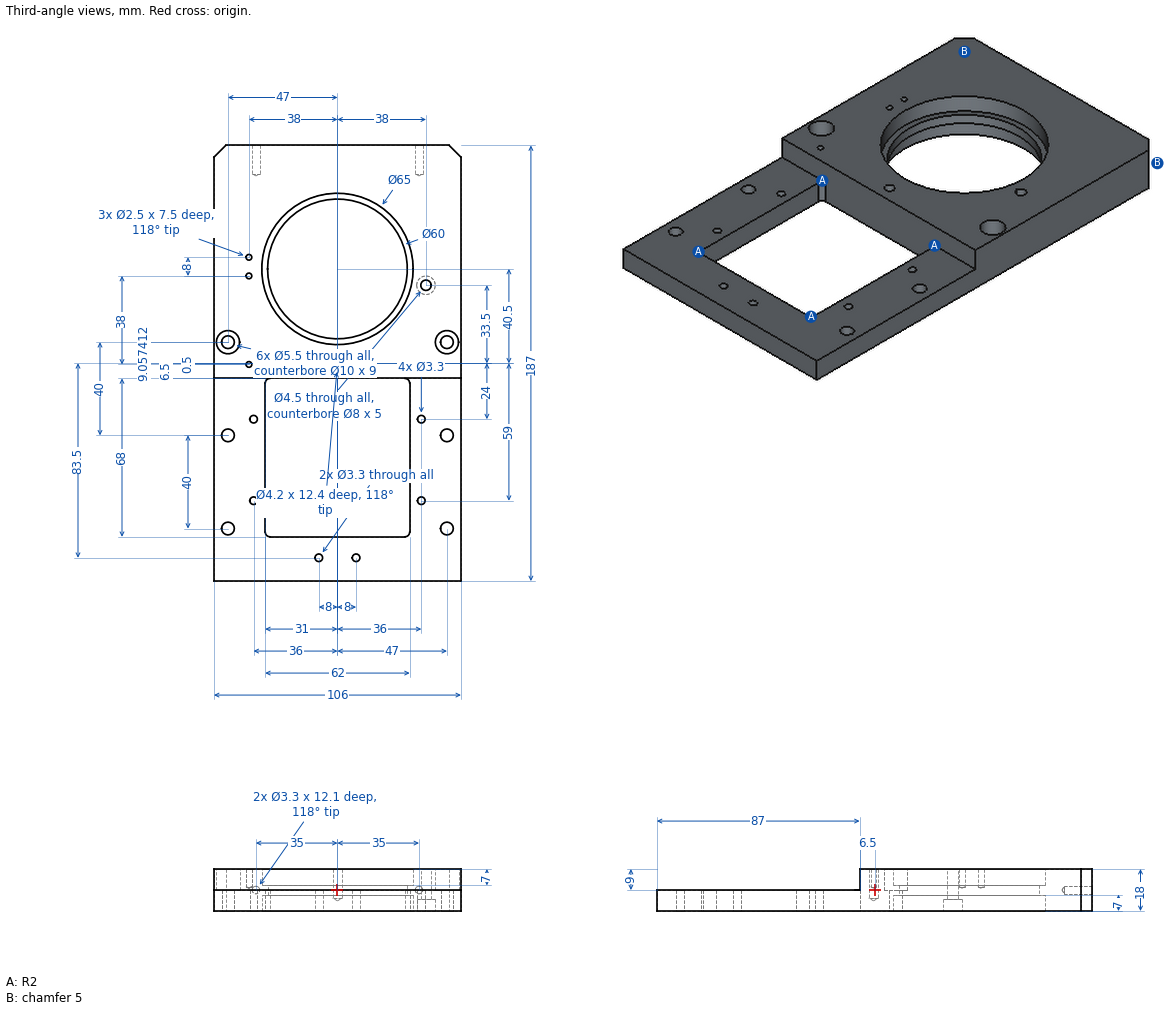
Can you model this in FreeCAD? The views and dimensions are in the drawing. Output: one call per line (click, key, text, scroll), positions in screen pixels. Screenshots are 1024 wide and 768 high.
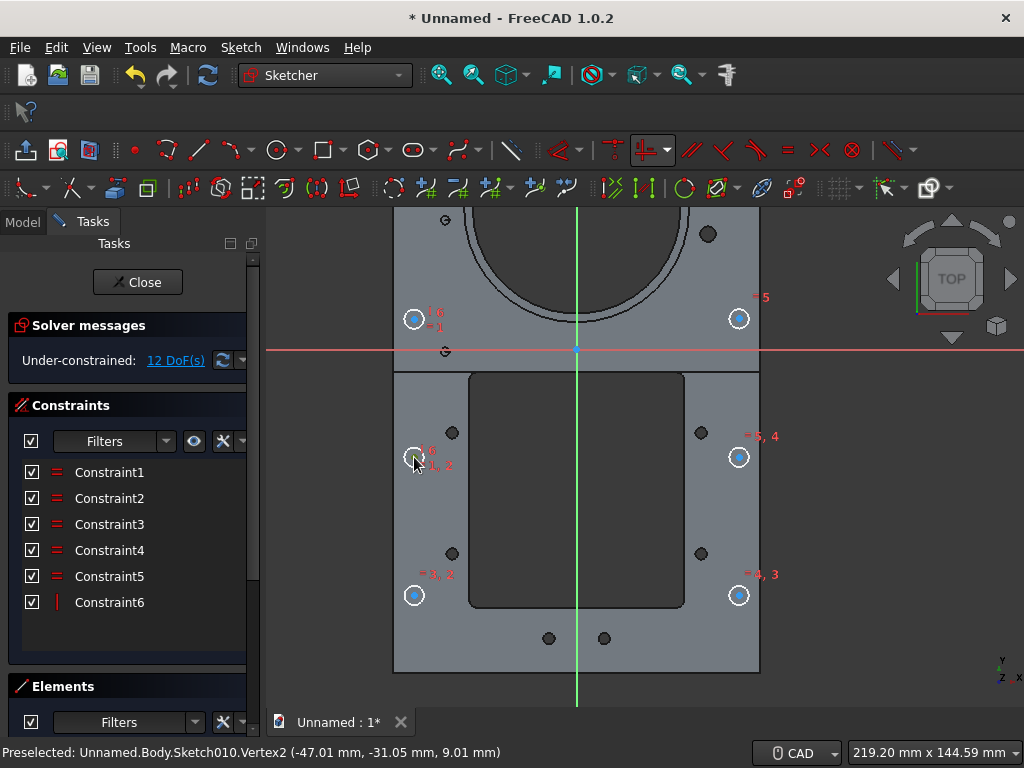
click(414, 595)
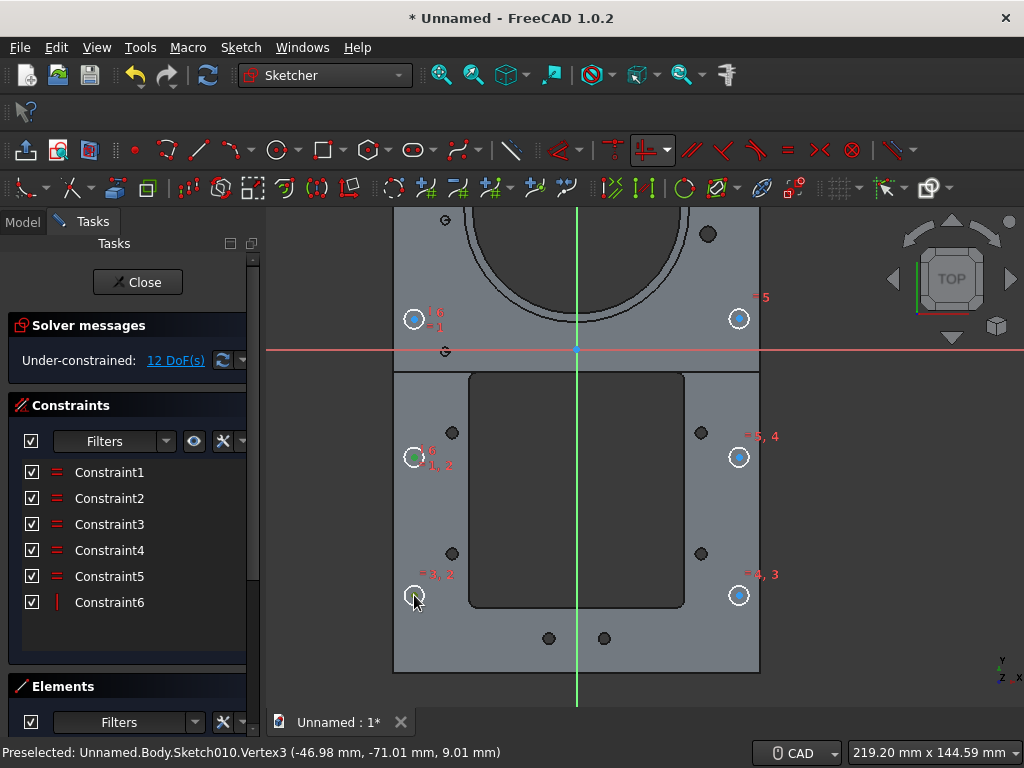
click(670, 150)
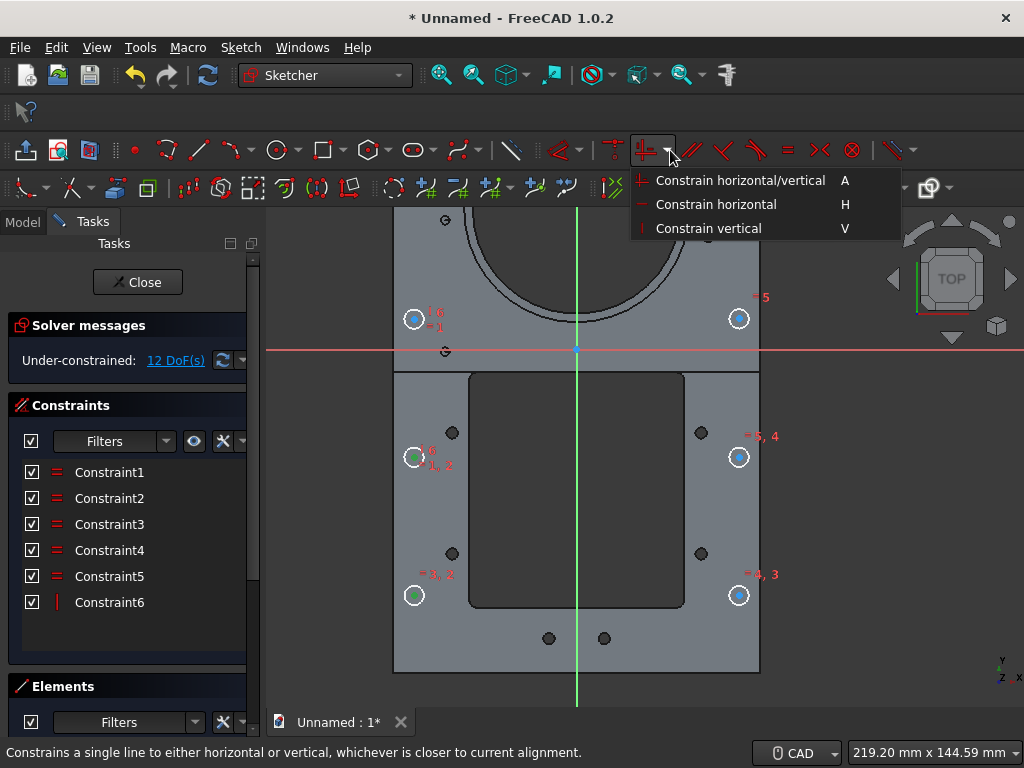
click(766, 228)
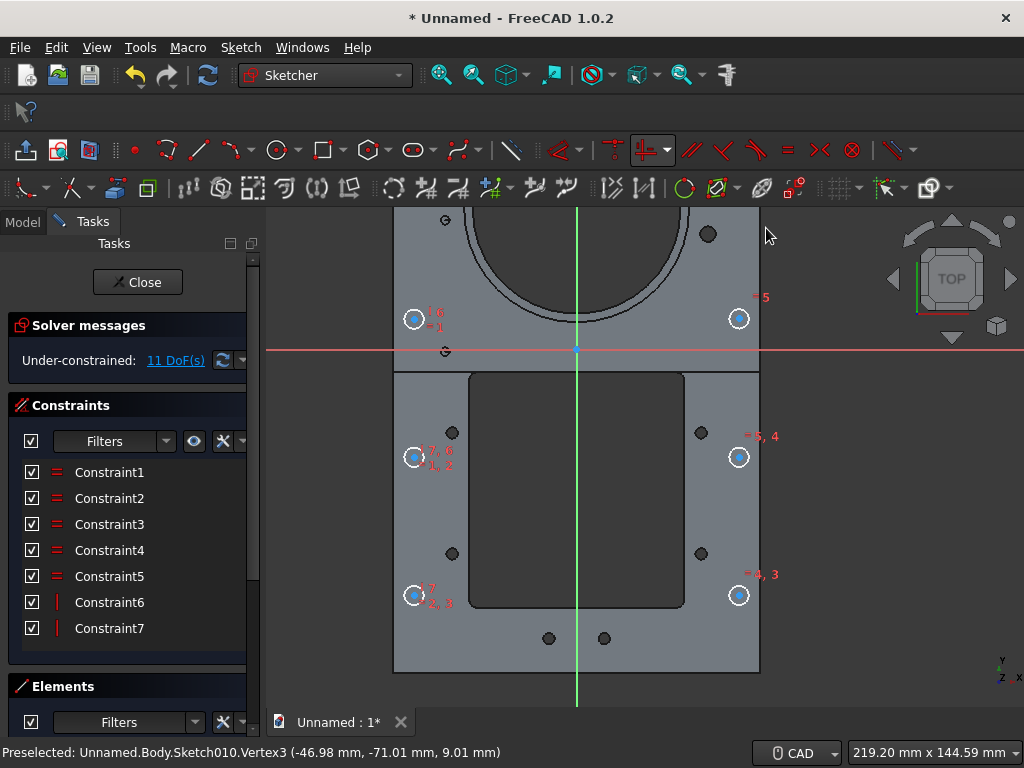
click(414, 595)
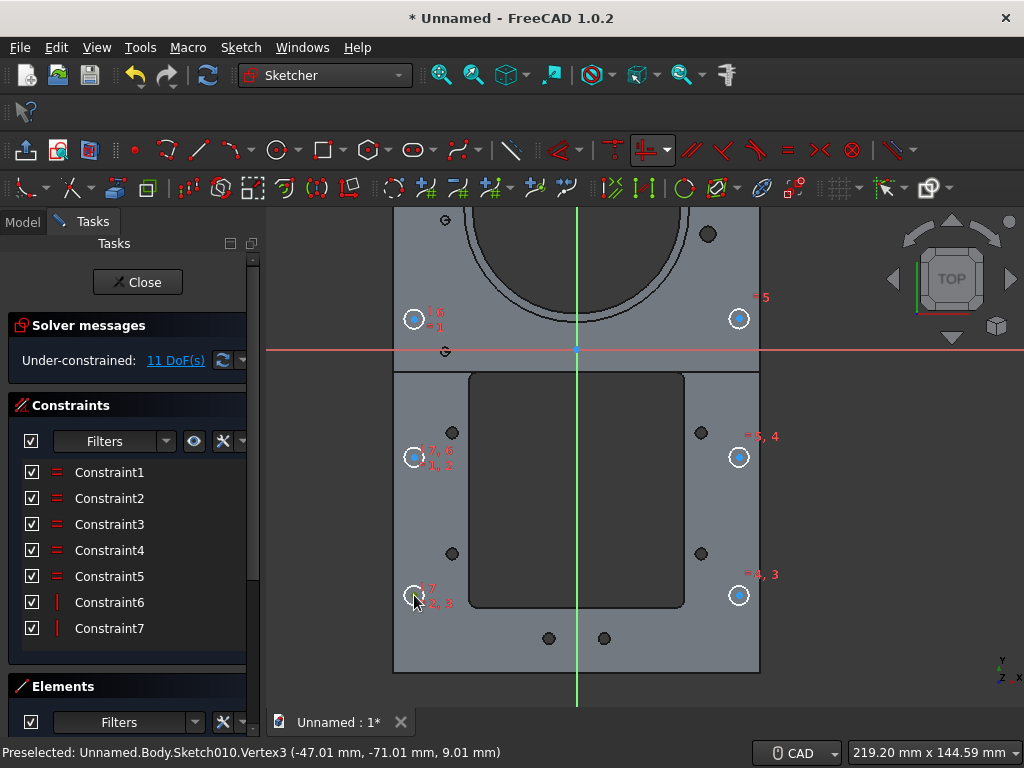
click(739, 595)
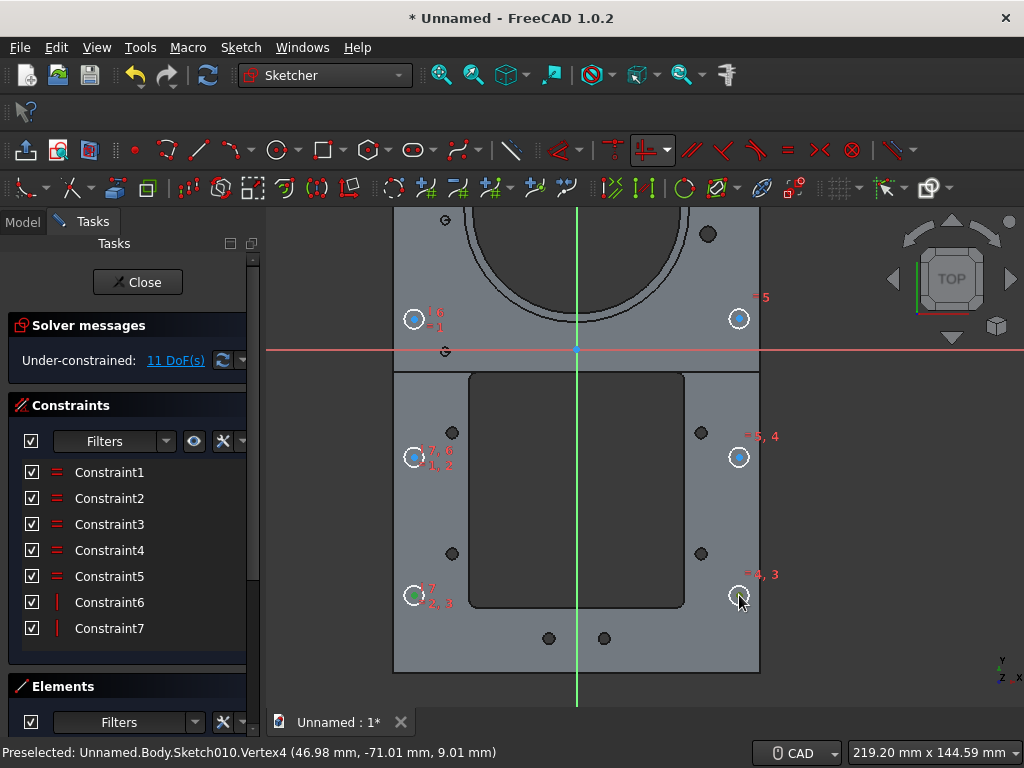
click(670, 150)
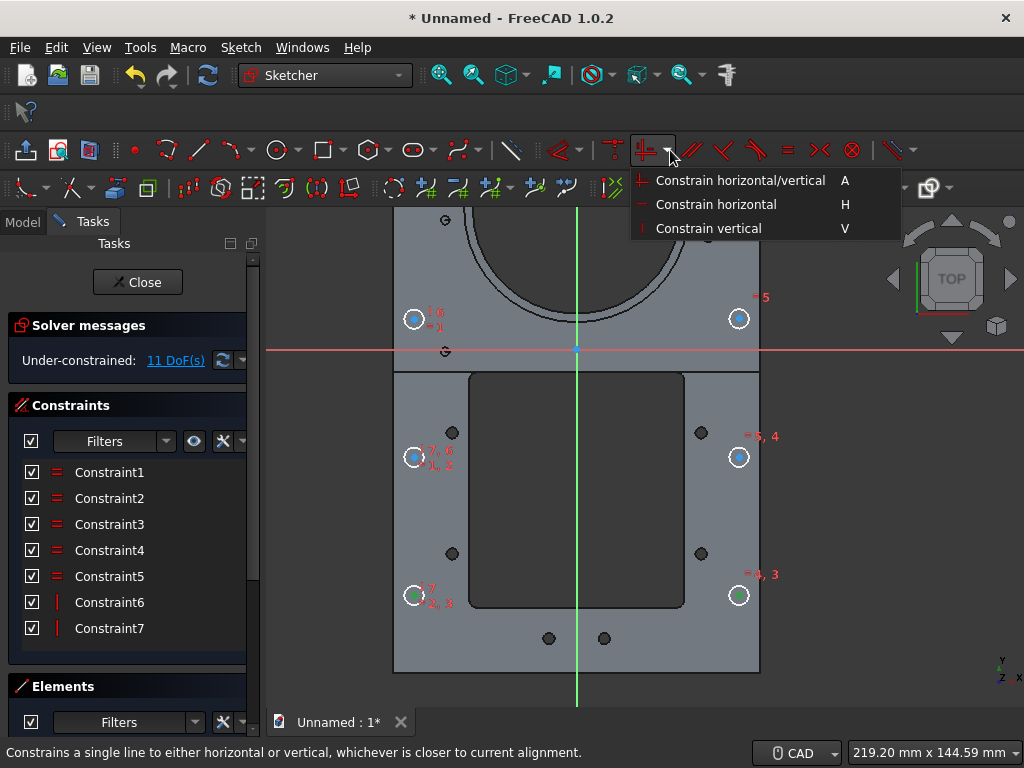
click(766, 204)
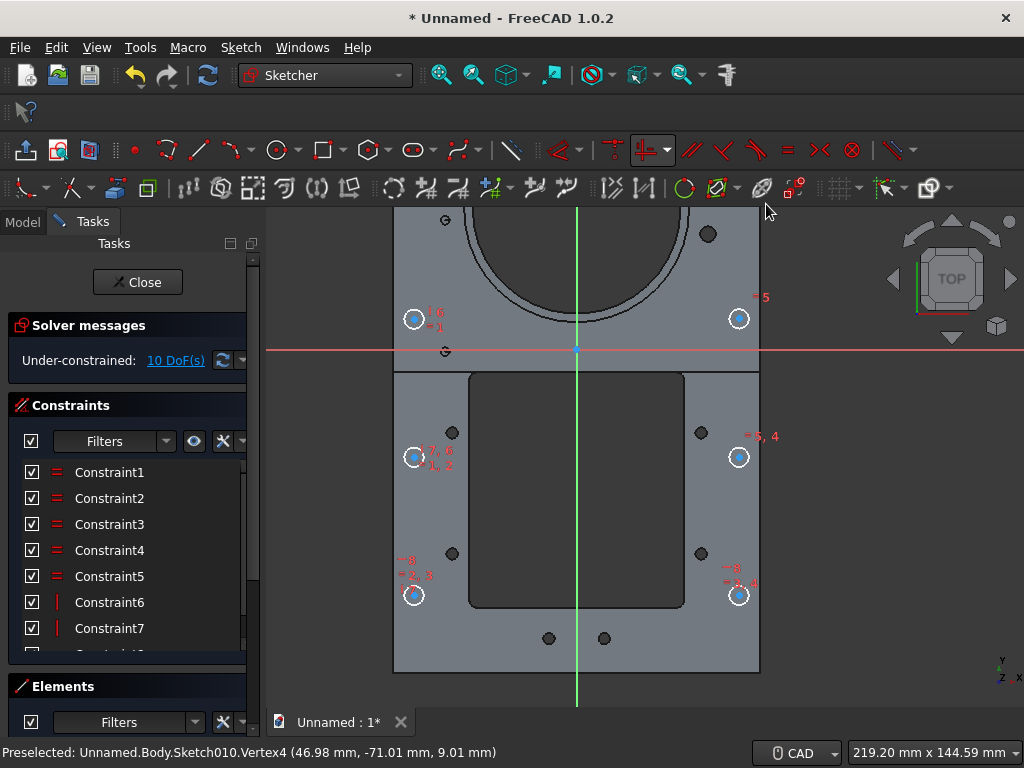
click(739, 595)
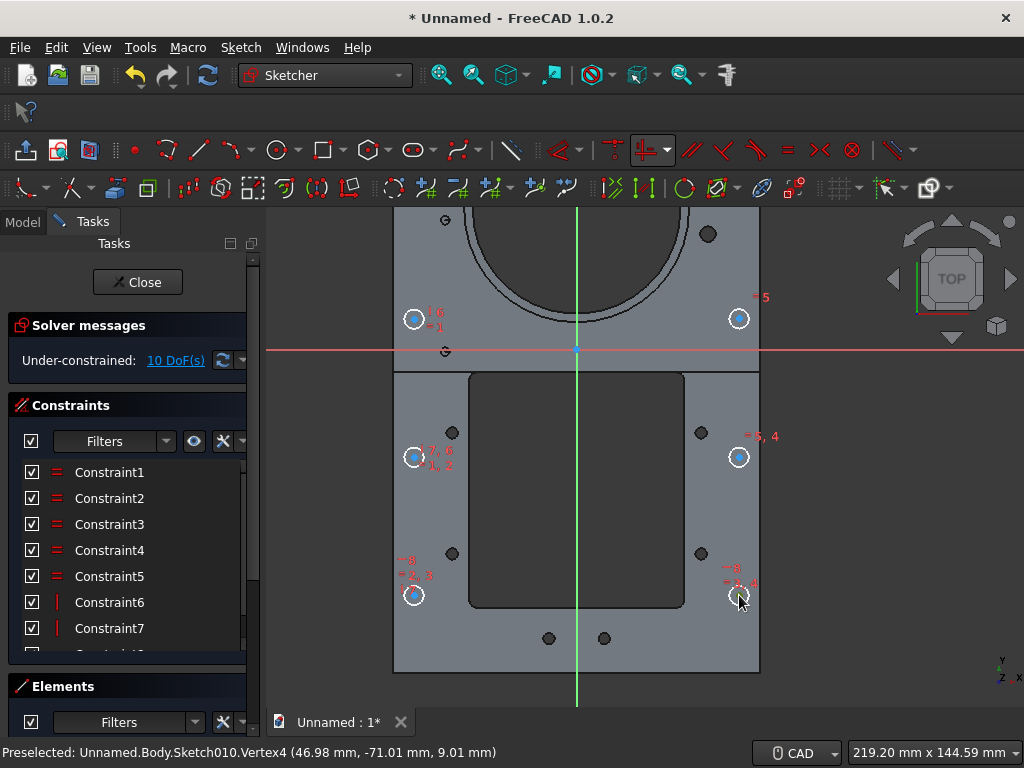
click(739, 457)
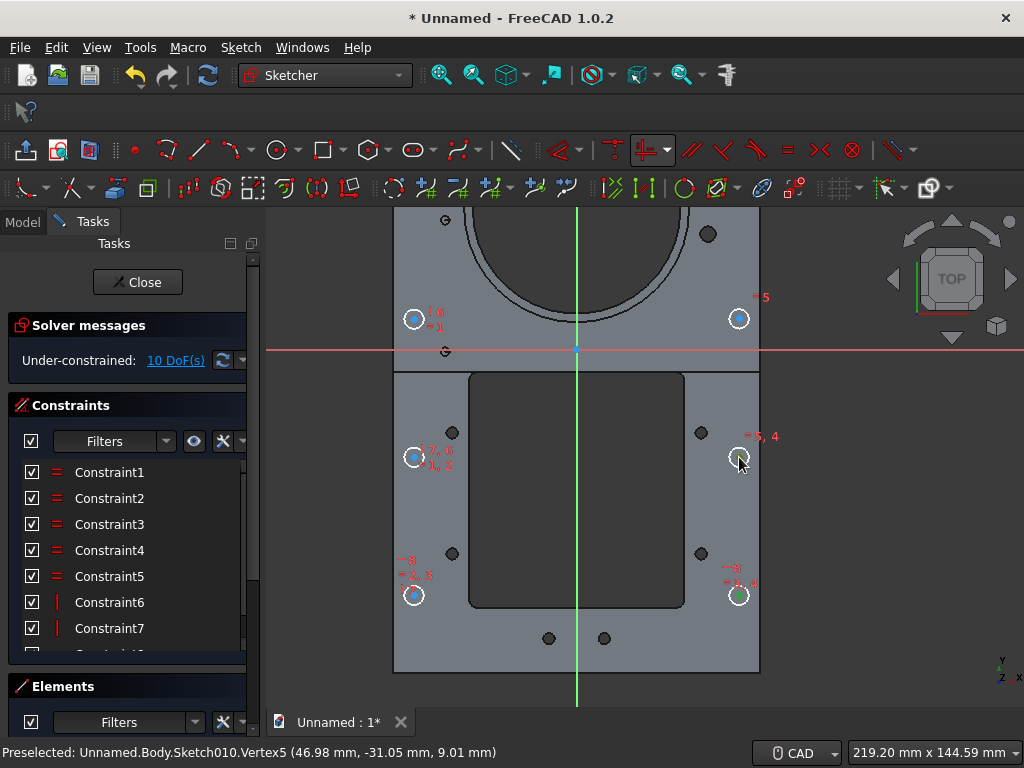
click(670, 150)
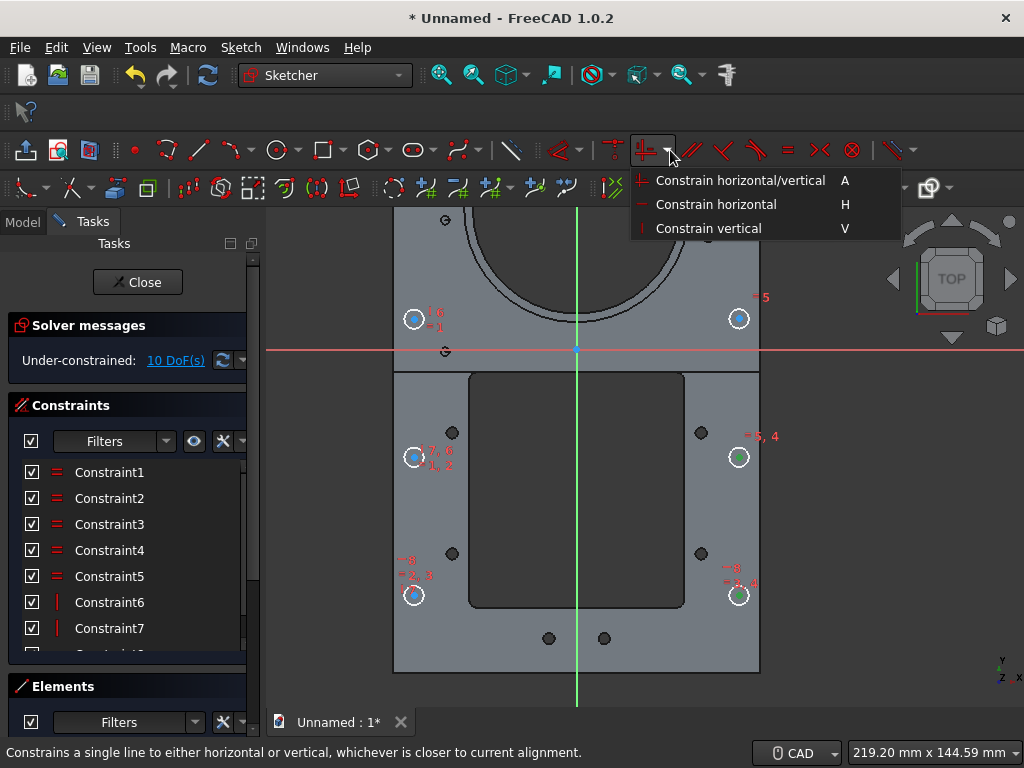
click(766, 228)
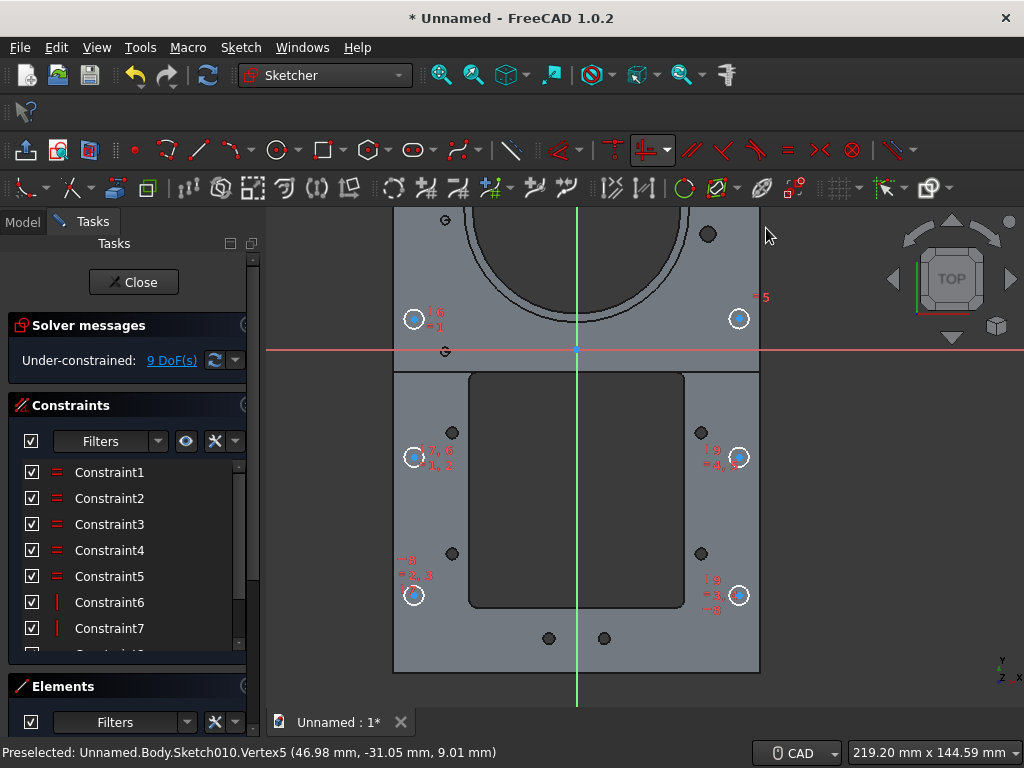
click(414, 457)